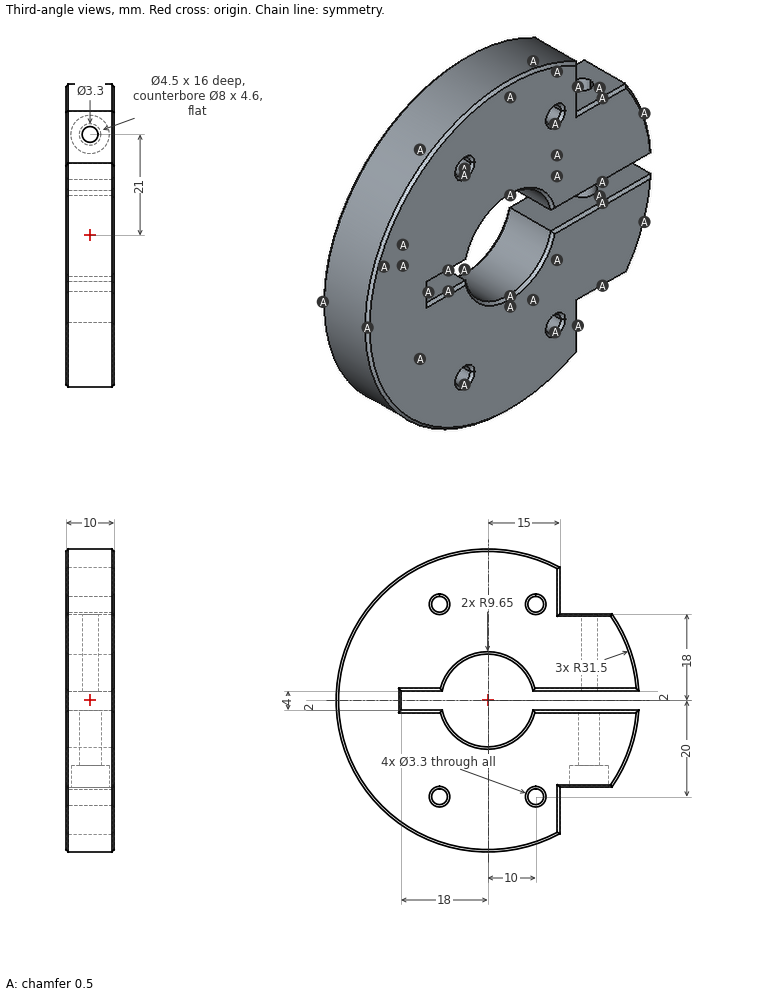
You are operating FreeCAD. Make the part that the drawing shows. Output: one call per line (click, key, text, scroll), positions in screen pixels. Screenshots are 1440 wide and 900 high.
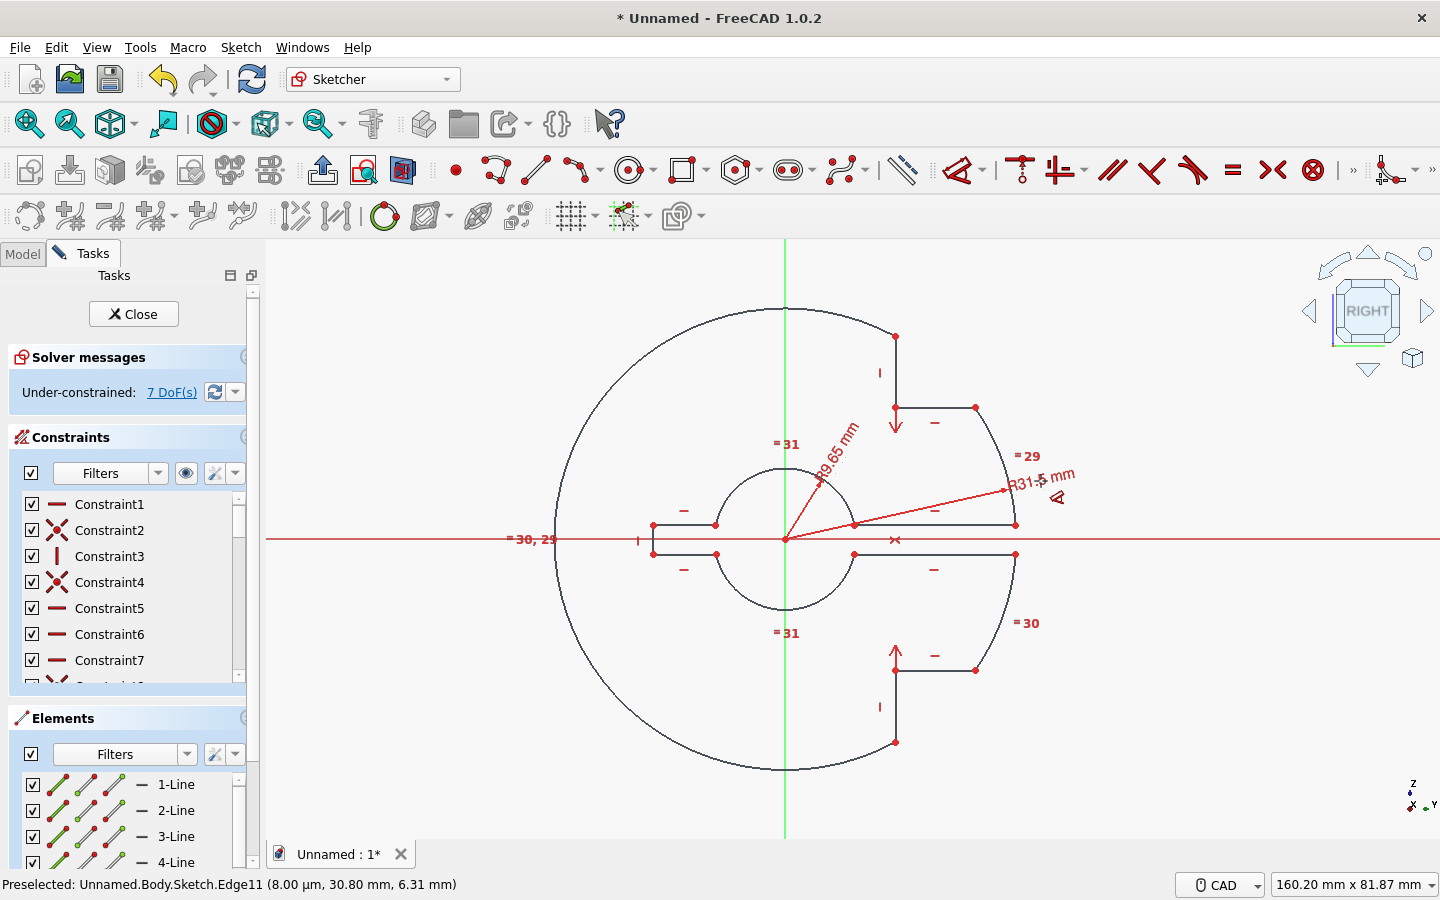
scroll(653, 543, up, 2)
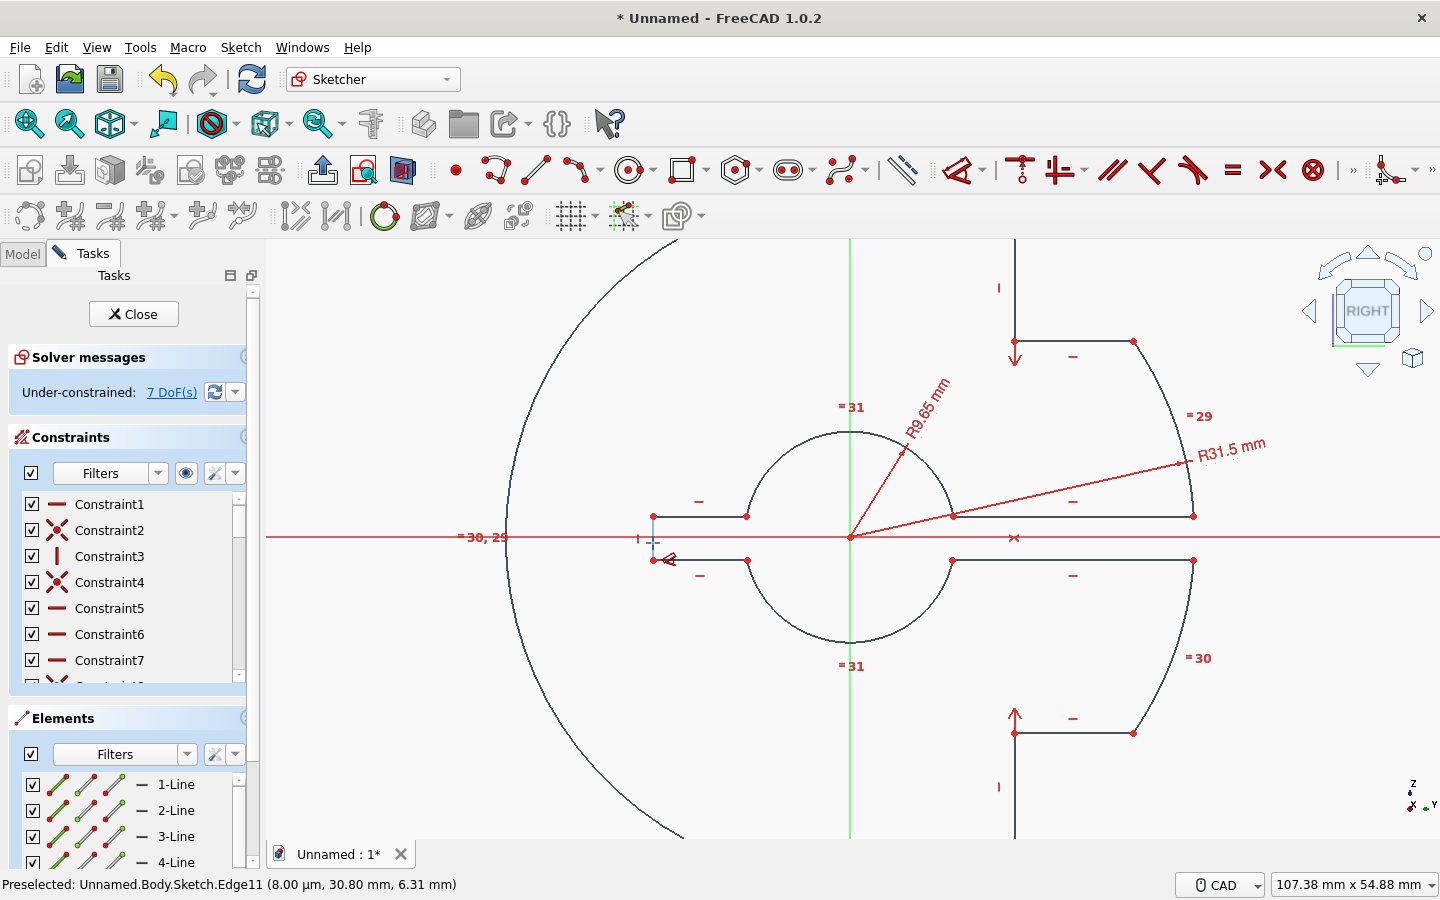
click(653, 543)
click(619, 523)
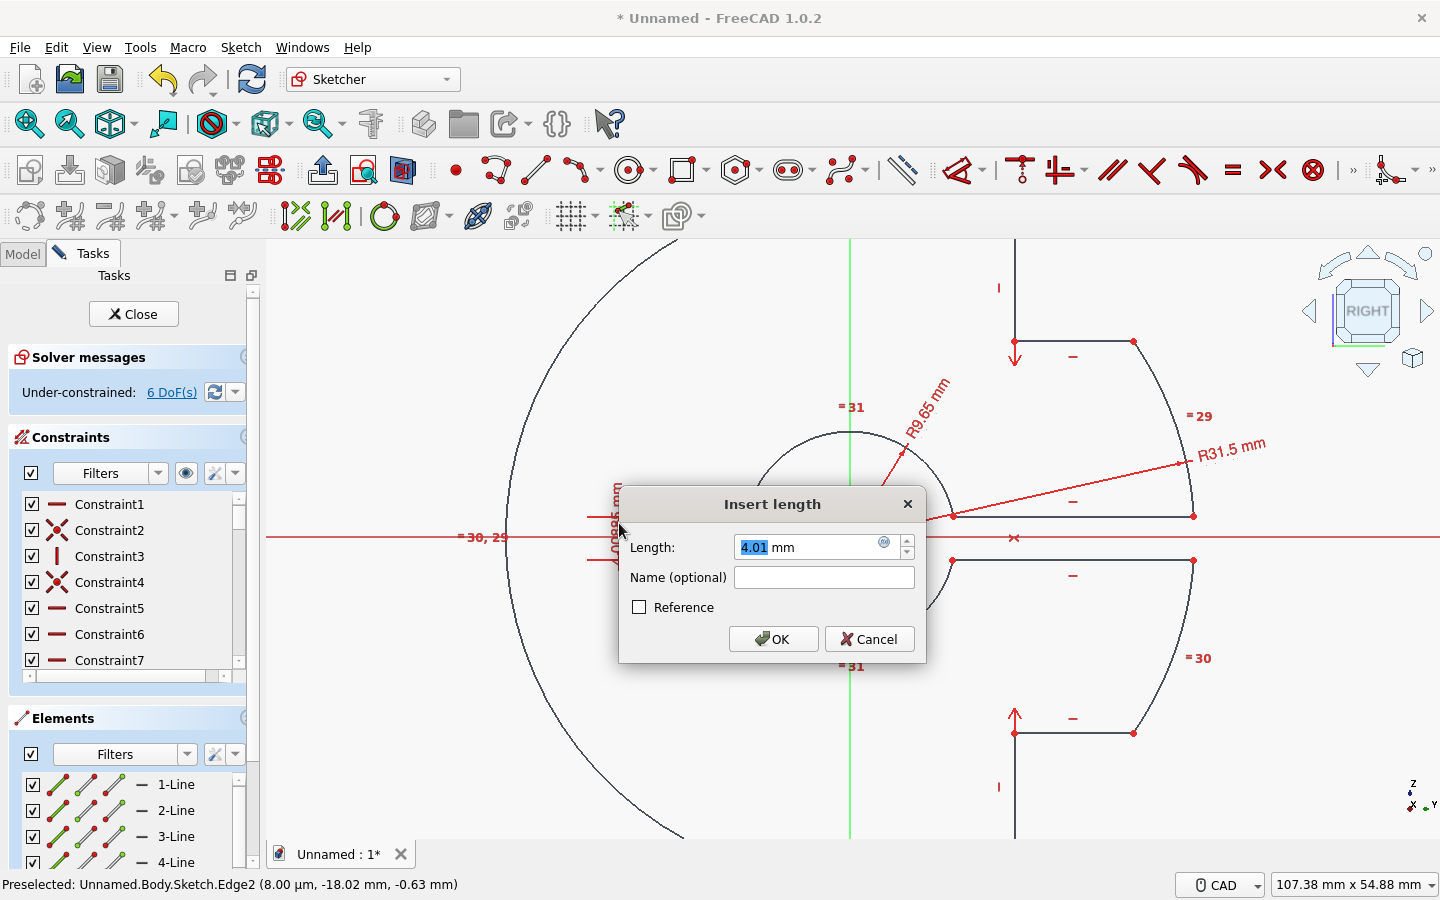
text(4)
key(Return)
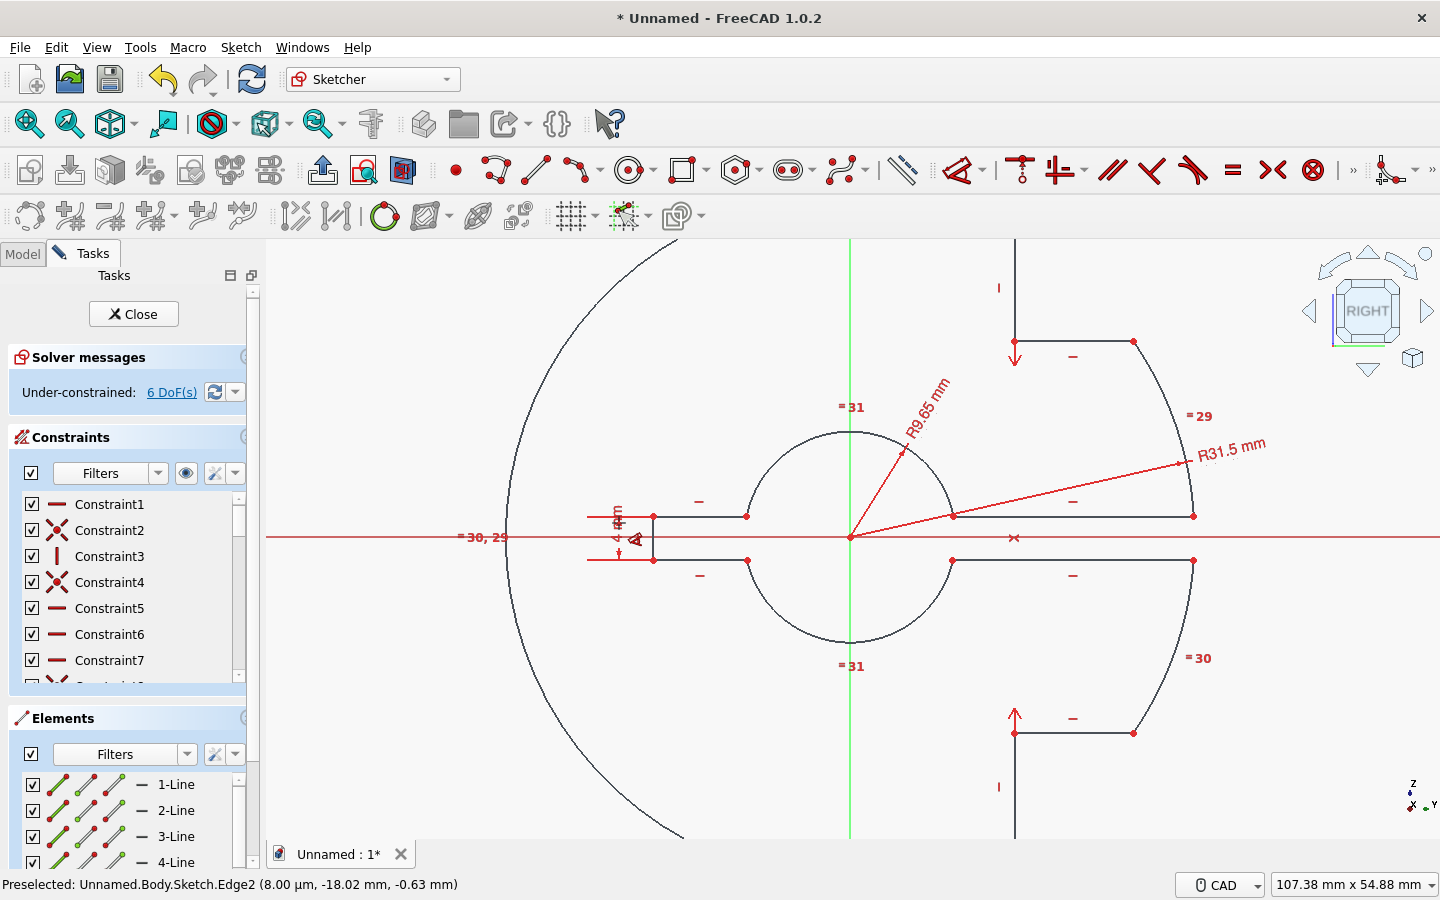
scroll(747, 560, up, 3)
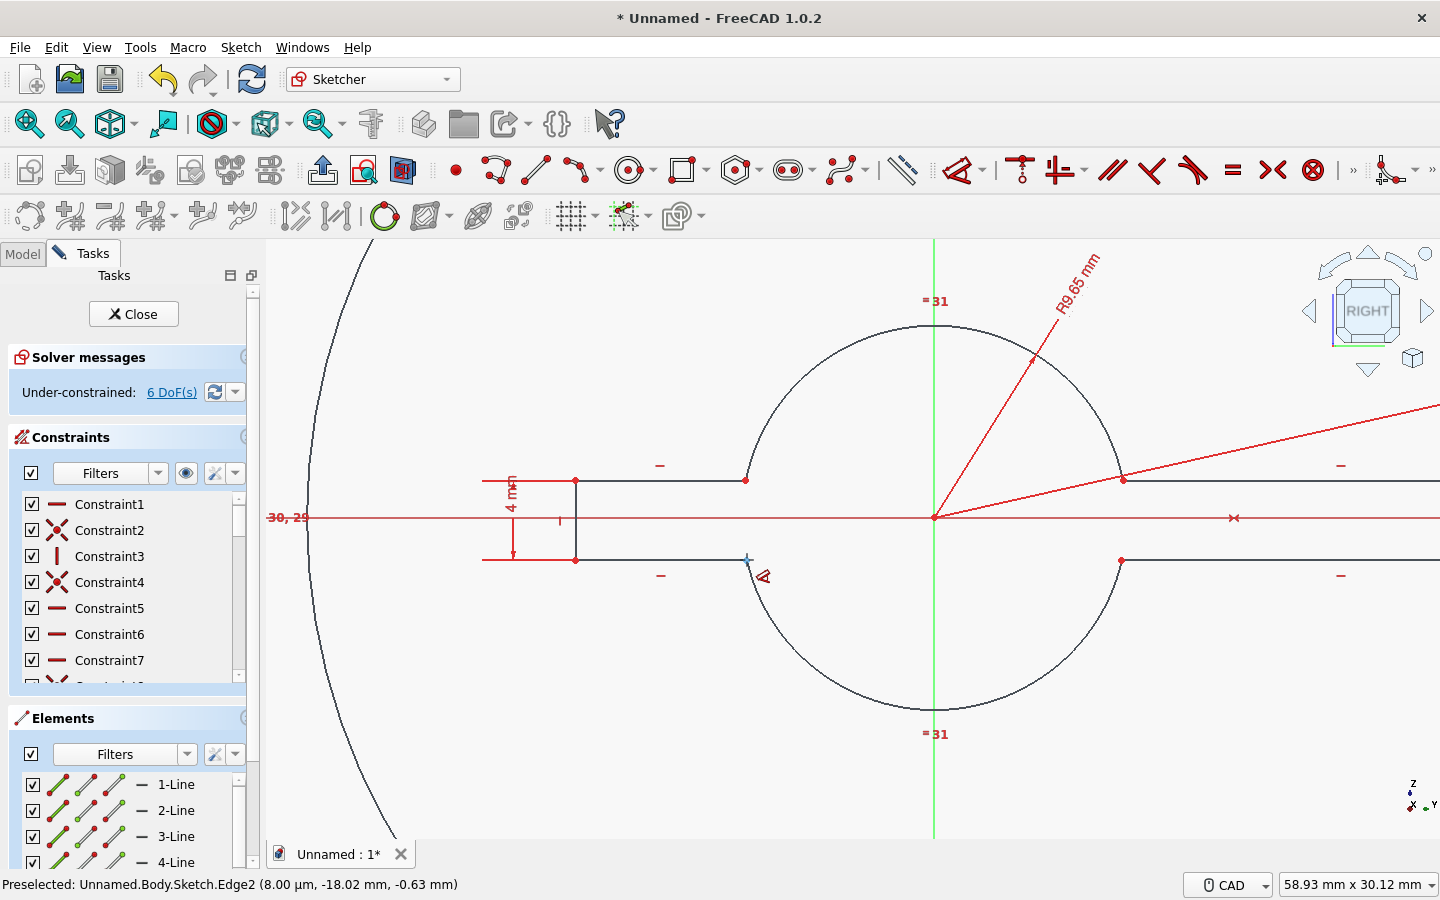
click(747, 560)
click(713, 539)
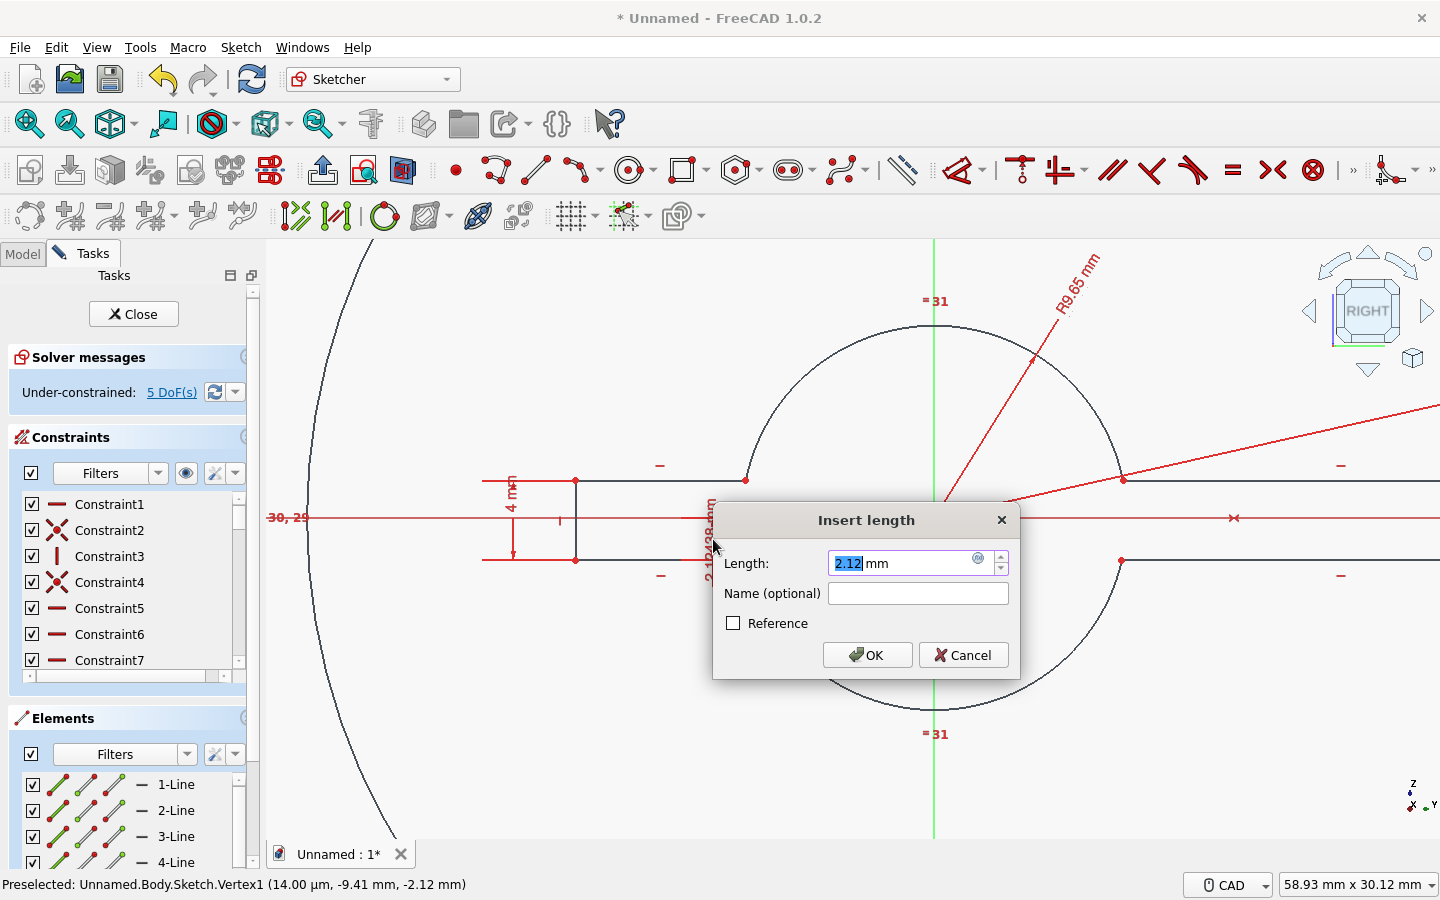
text(2)
key(Return)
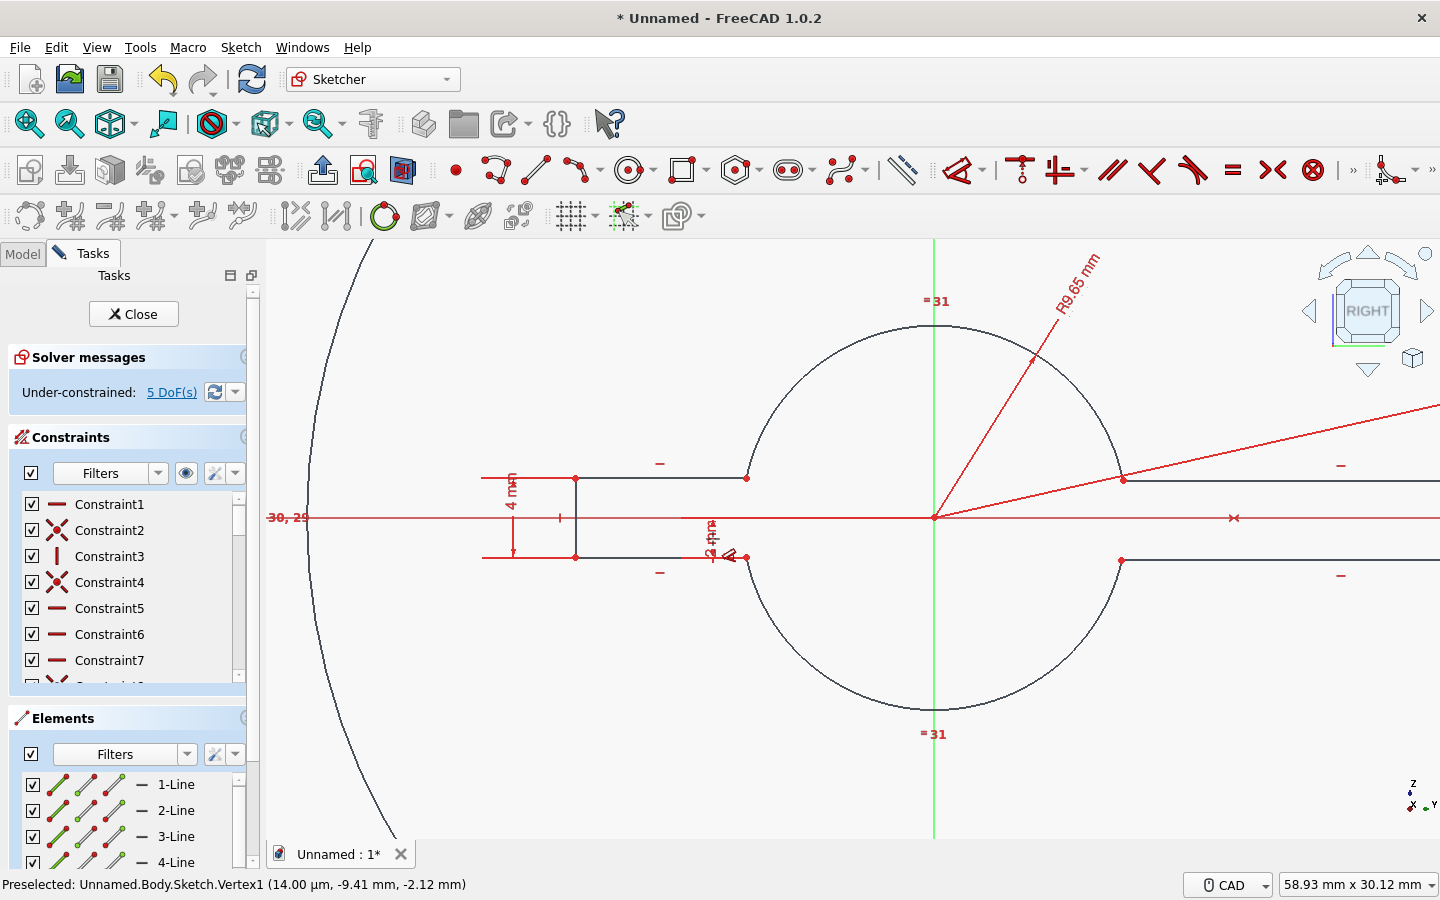
click(1123, 481)
click(1157, 499)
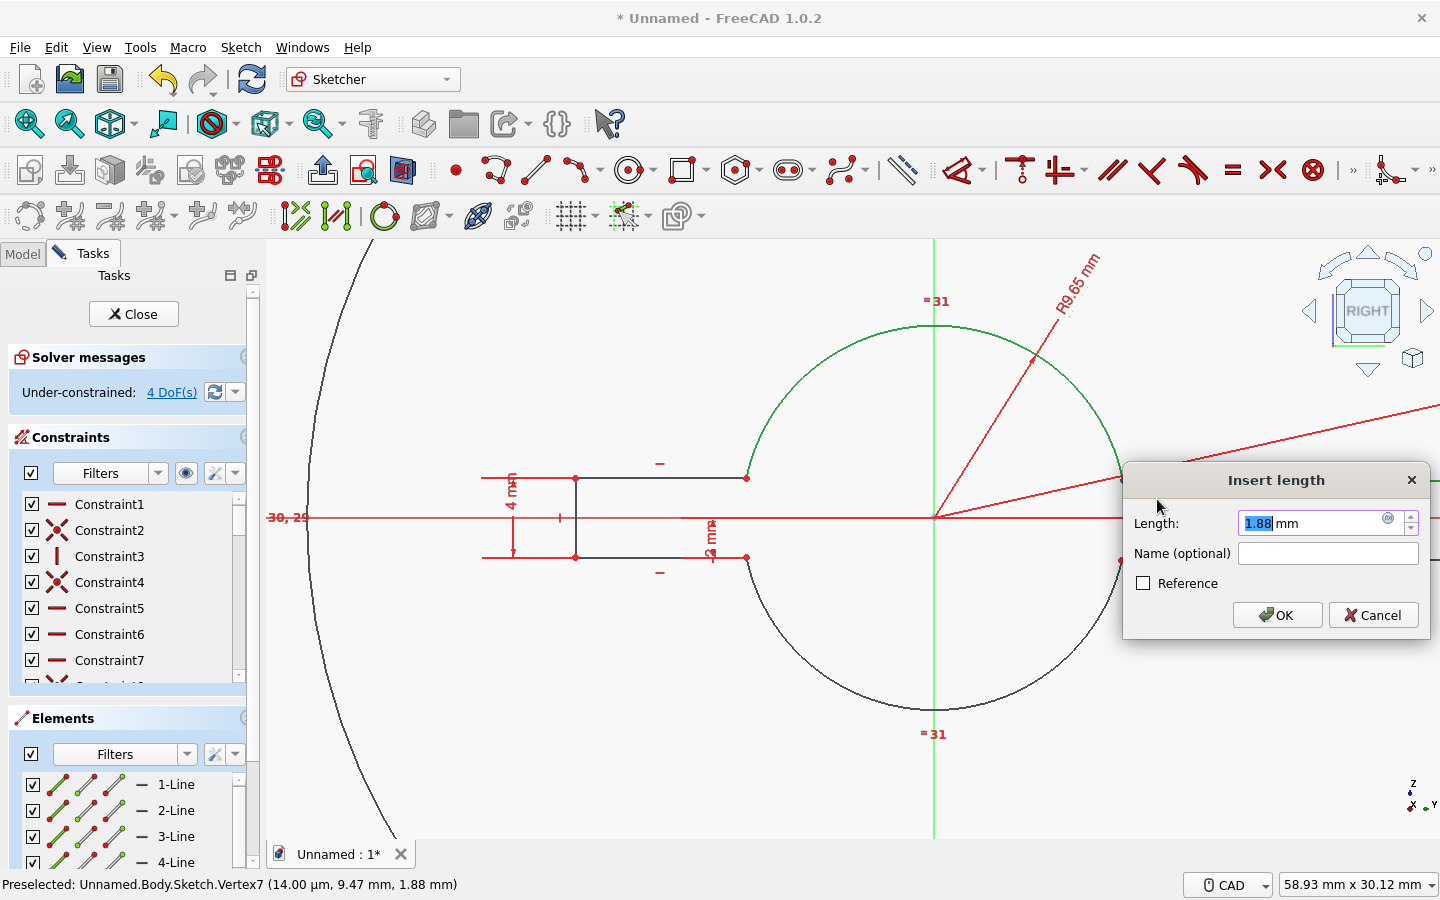
text(2)
key(Return)